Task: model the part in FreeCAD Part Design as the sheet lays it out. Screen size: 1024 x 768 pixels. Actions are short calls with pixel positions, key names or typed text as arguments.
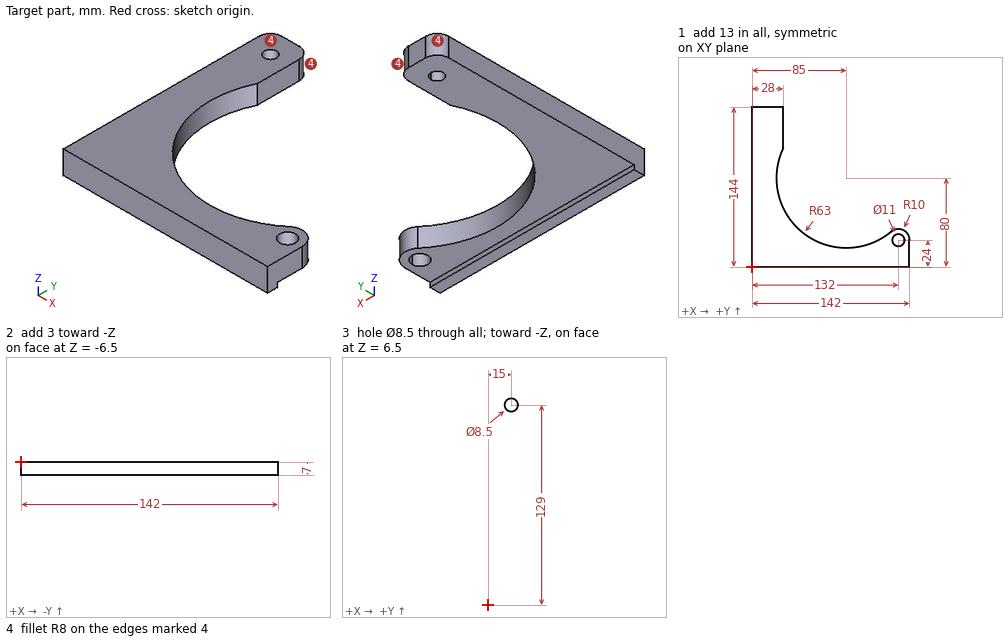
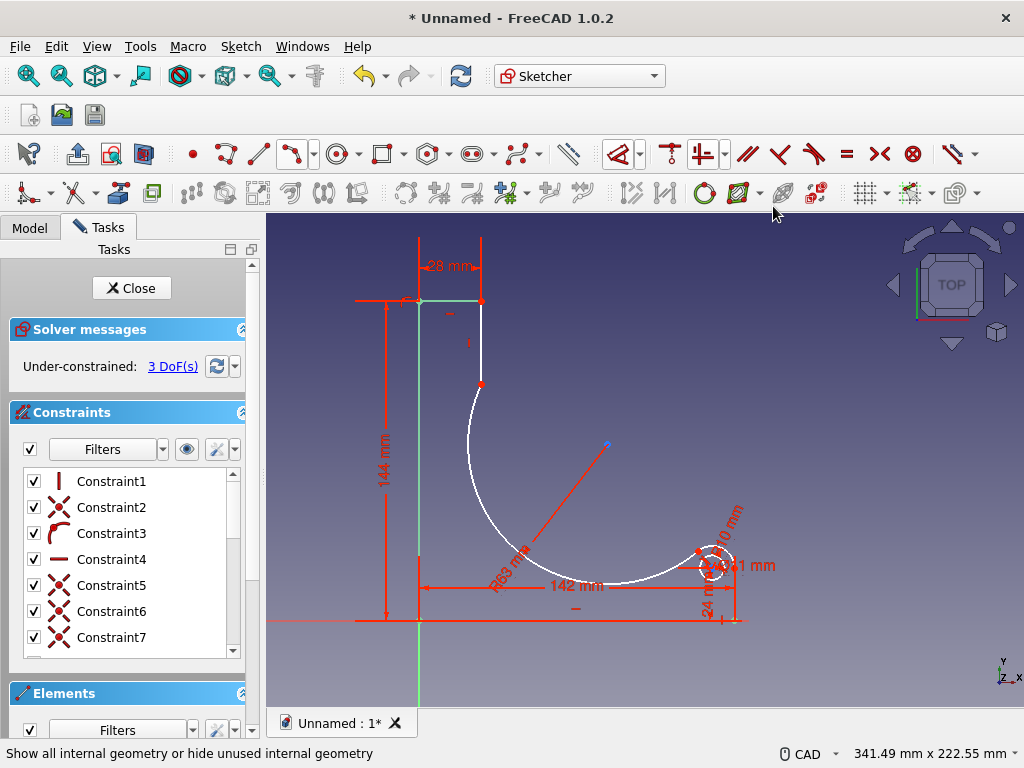
click(608, 444)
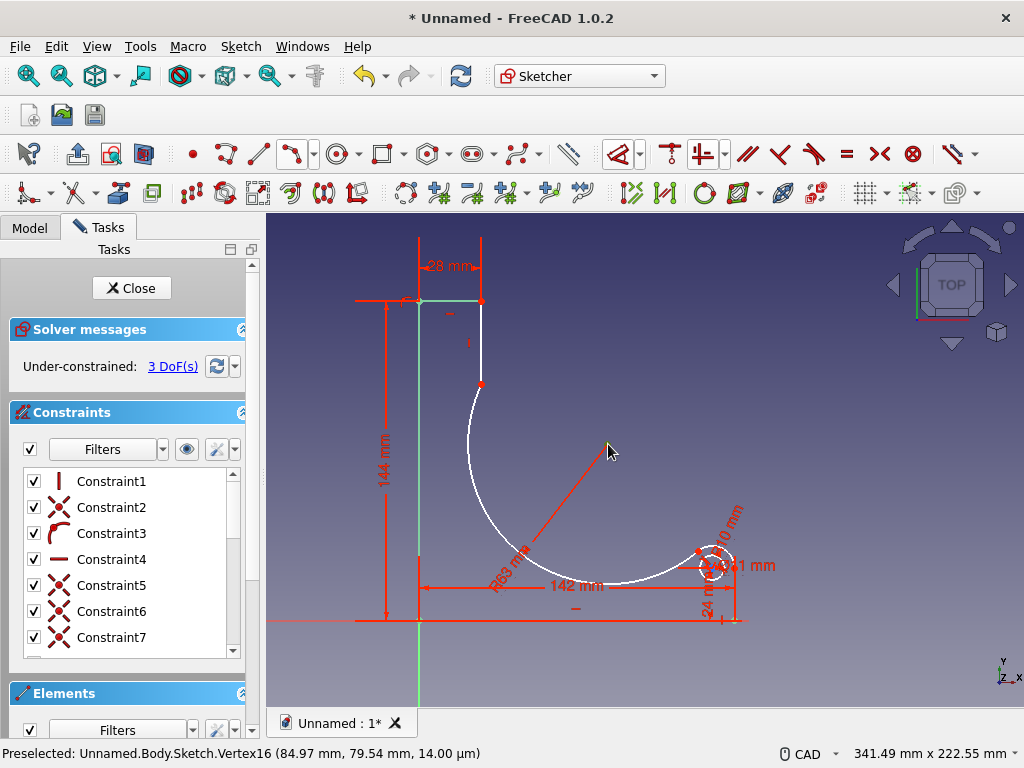
click(640, 154)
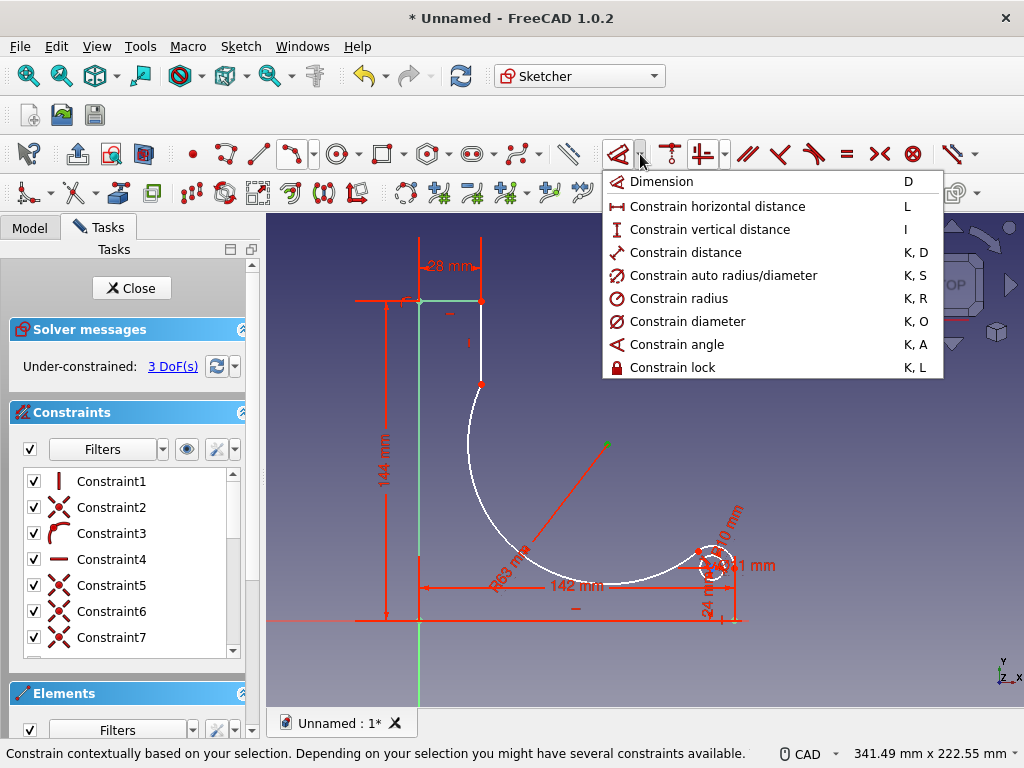
click(773, 206)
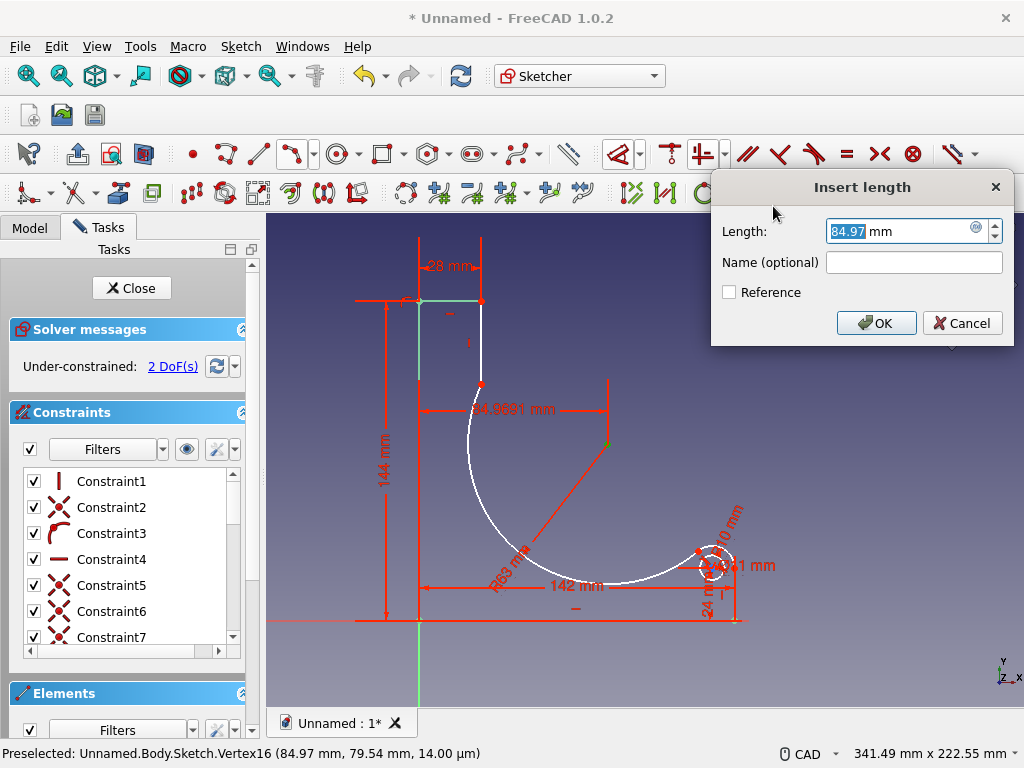
text(85)
key(Return)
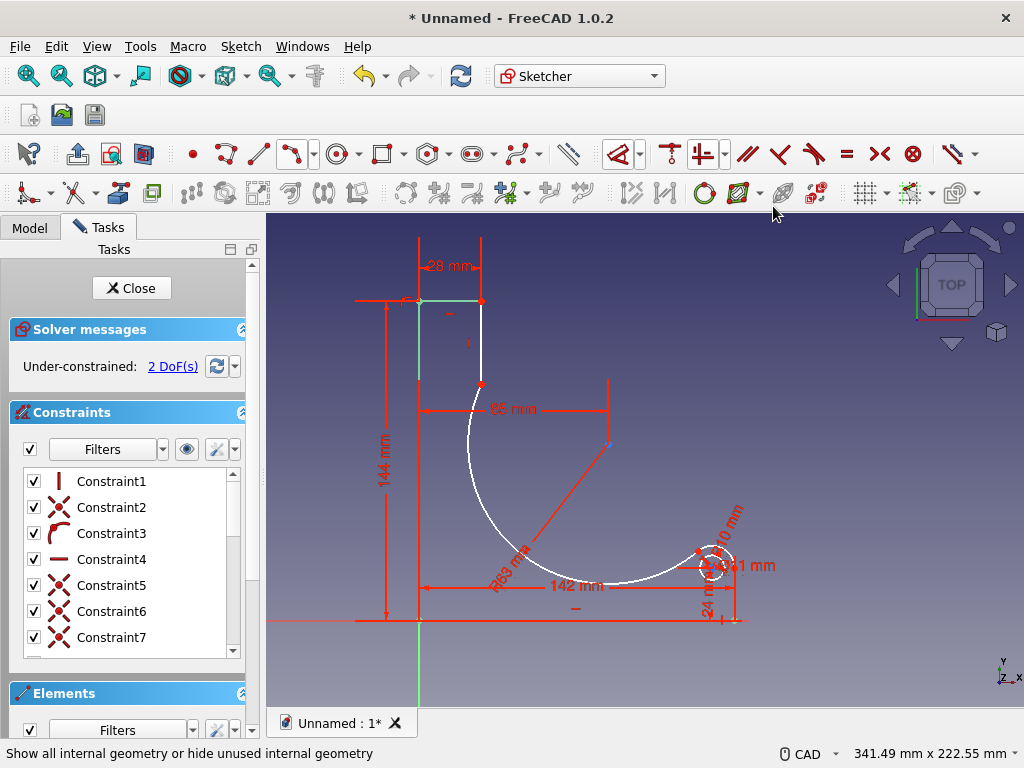
click(608, 444)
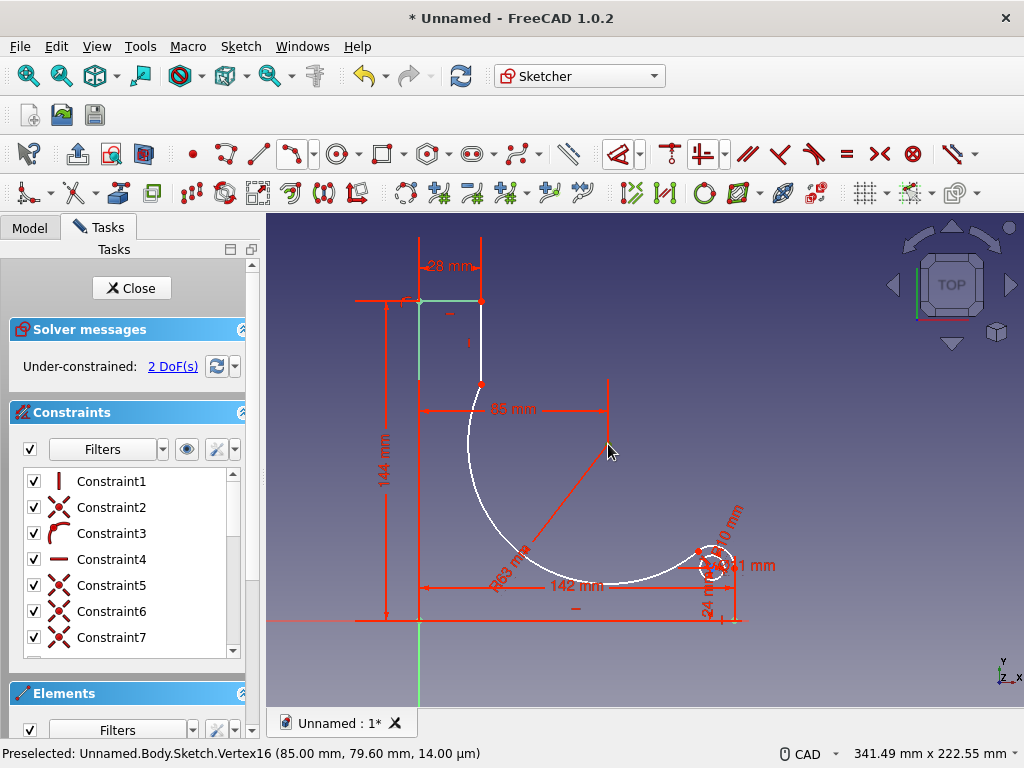
key(i)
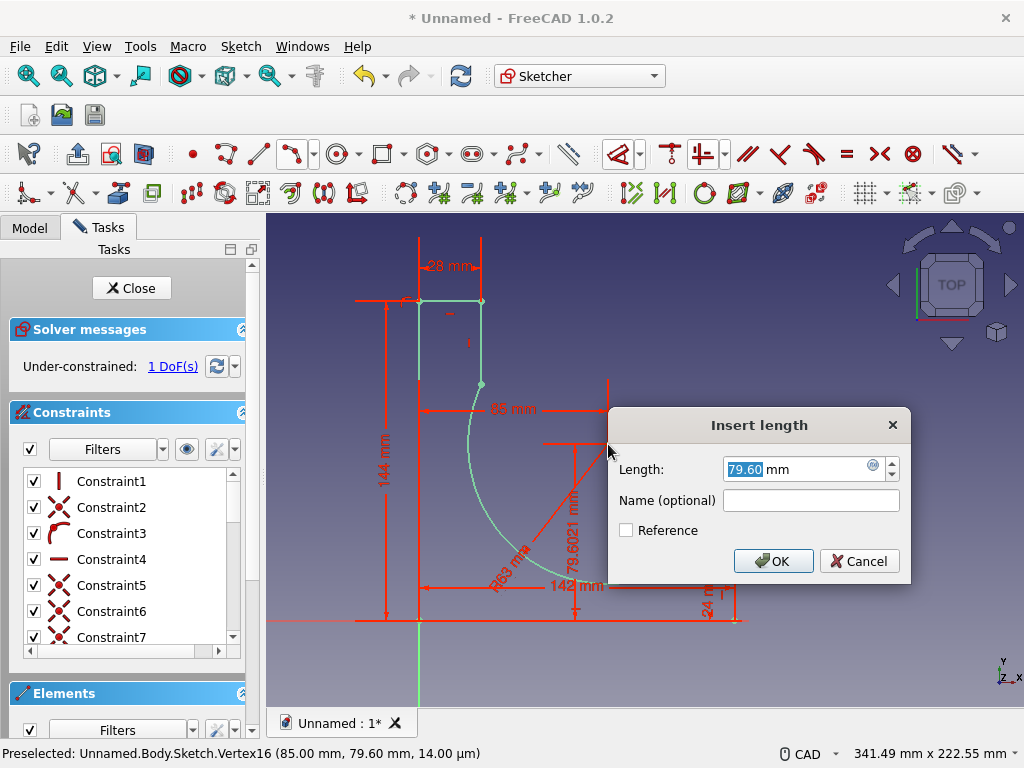
text(80)
key(Return)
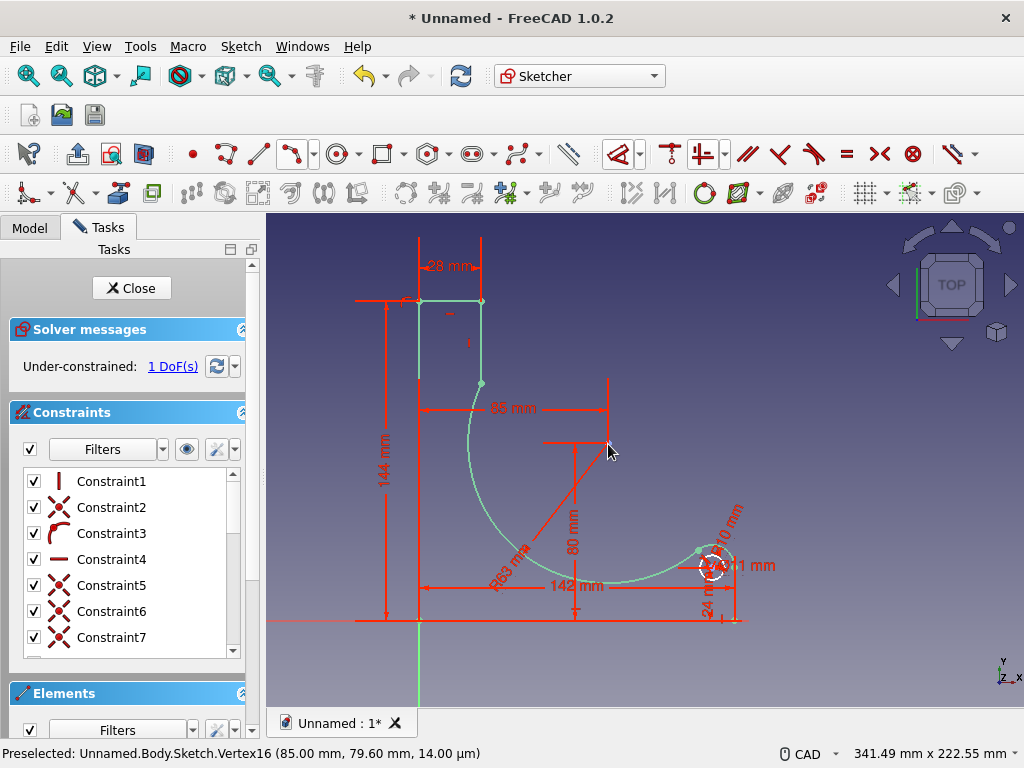
scroll(712, 568, up, 13)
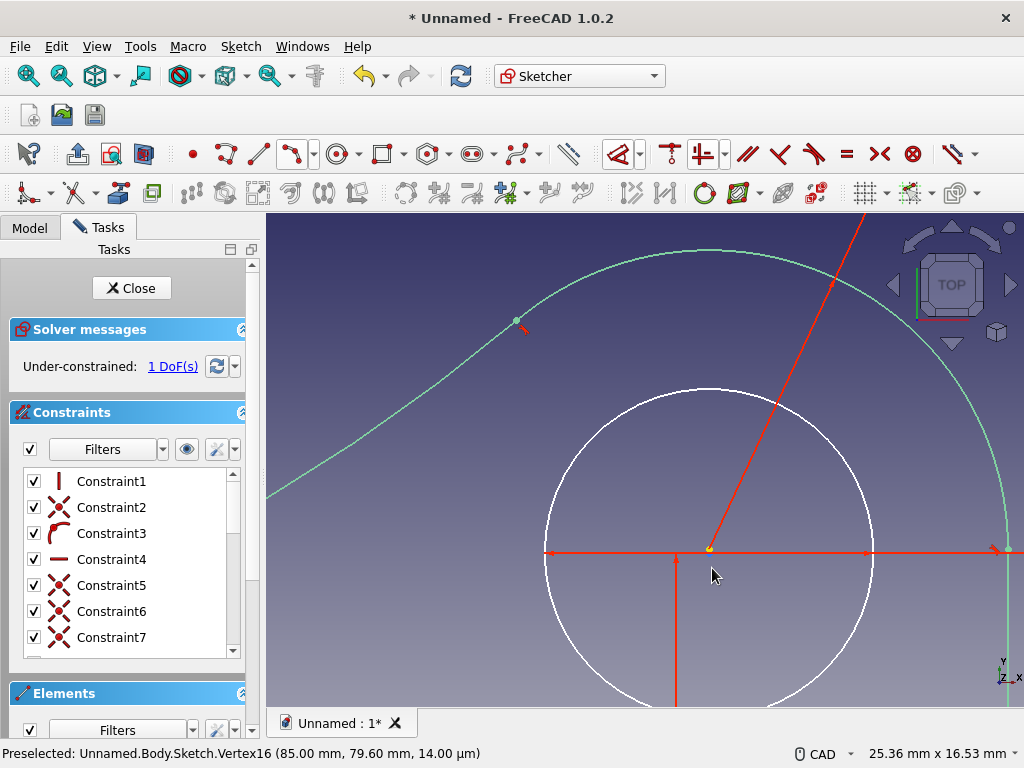
click(709, 553)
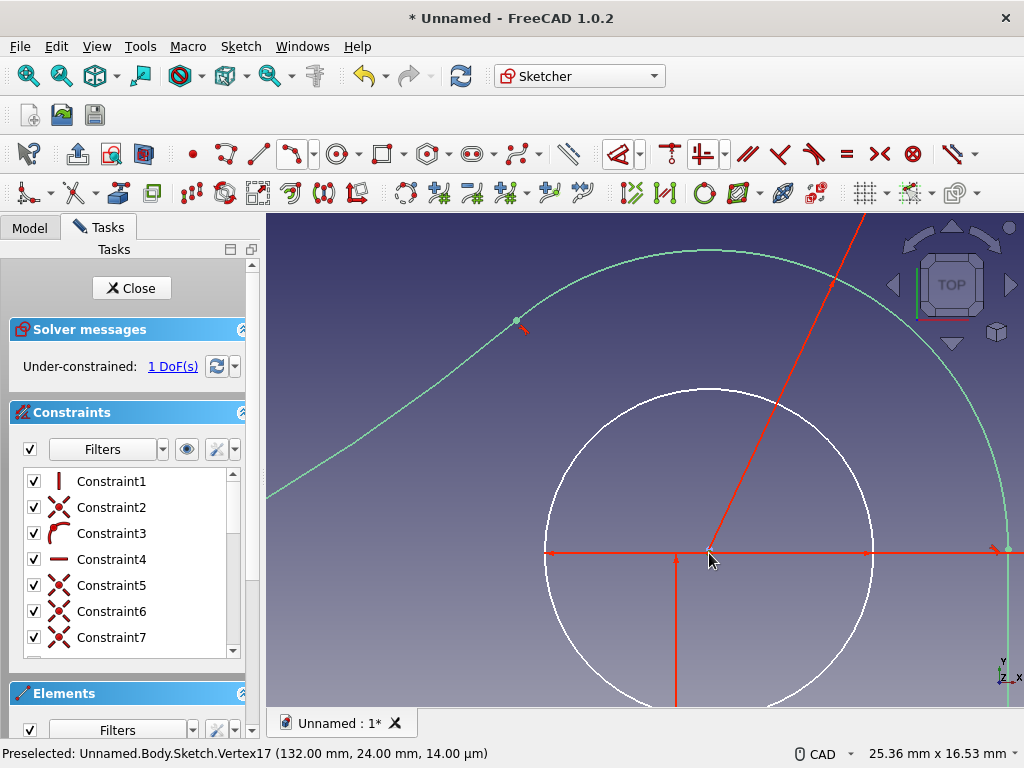
click(640, 154)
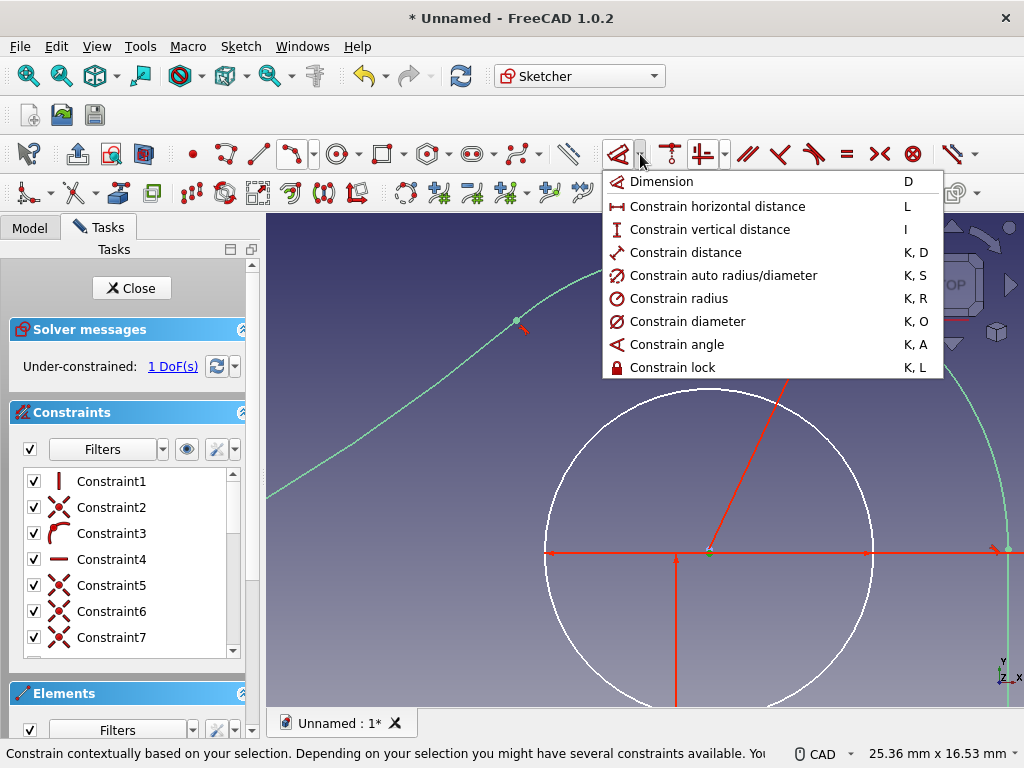
click(773, 206)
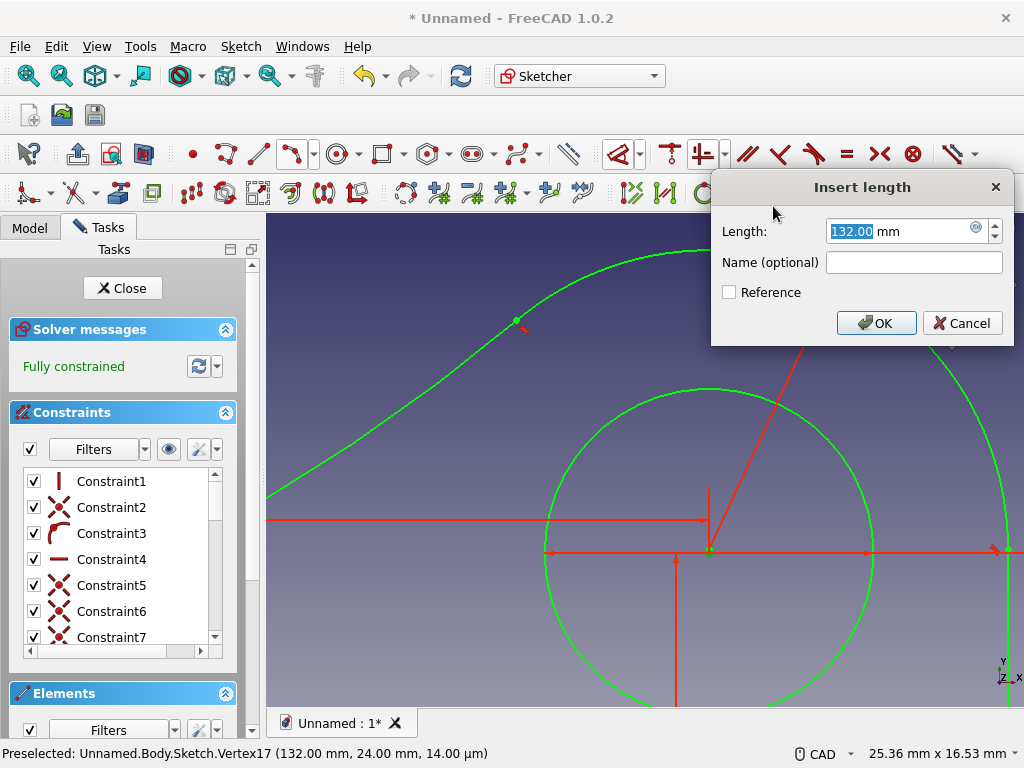
text(132)
key(Return)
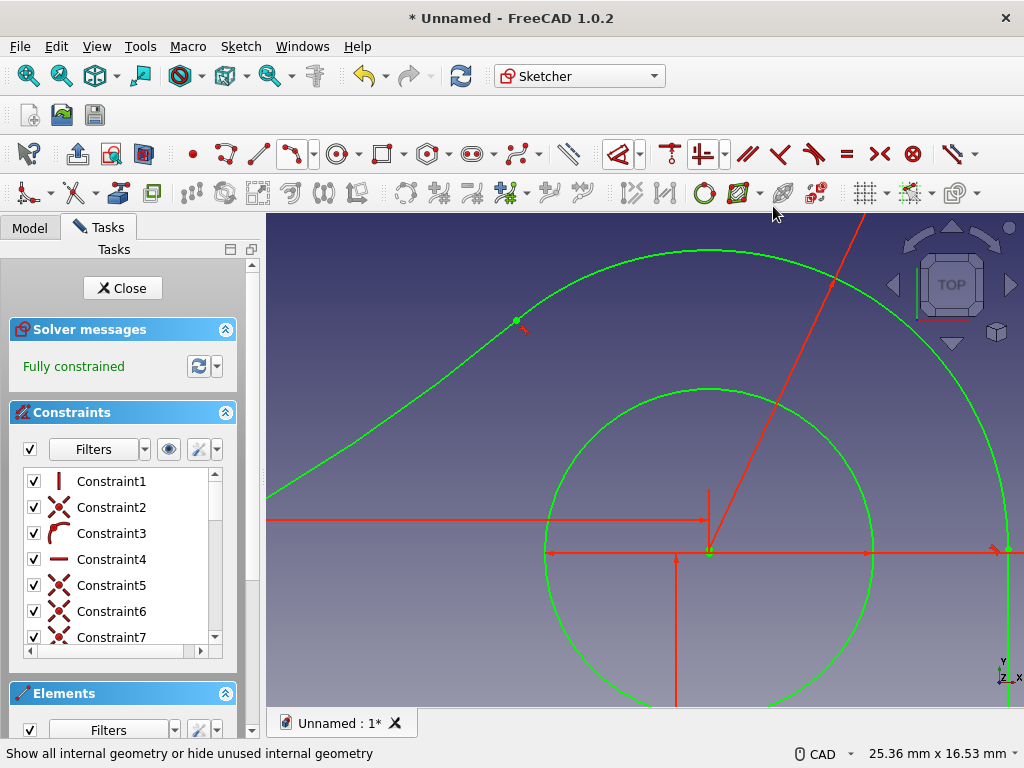
click(123, 288)